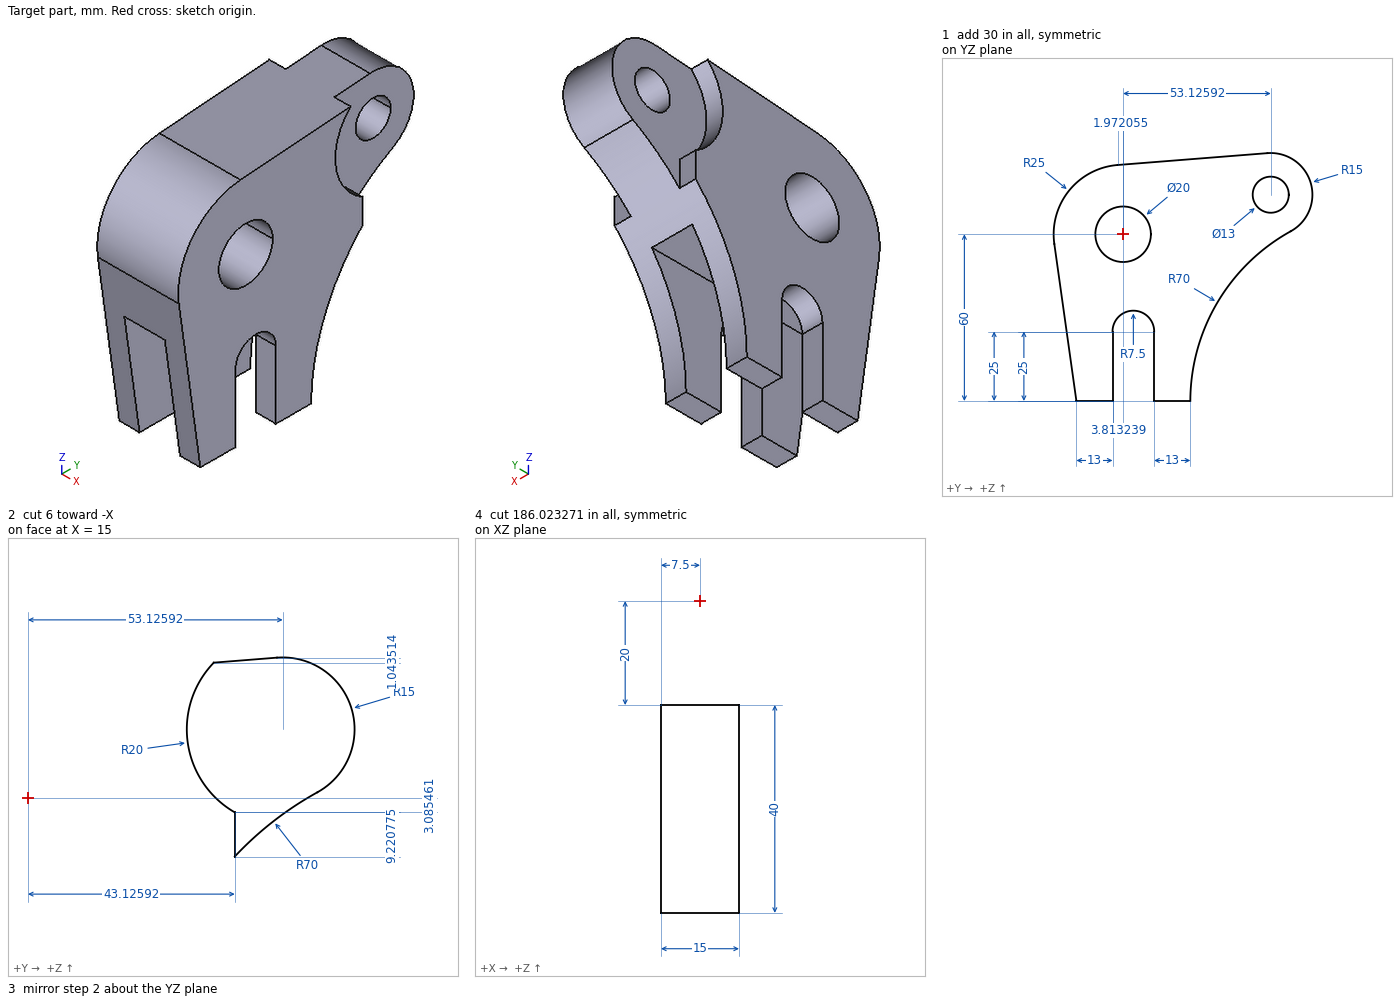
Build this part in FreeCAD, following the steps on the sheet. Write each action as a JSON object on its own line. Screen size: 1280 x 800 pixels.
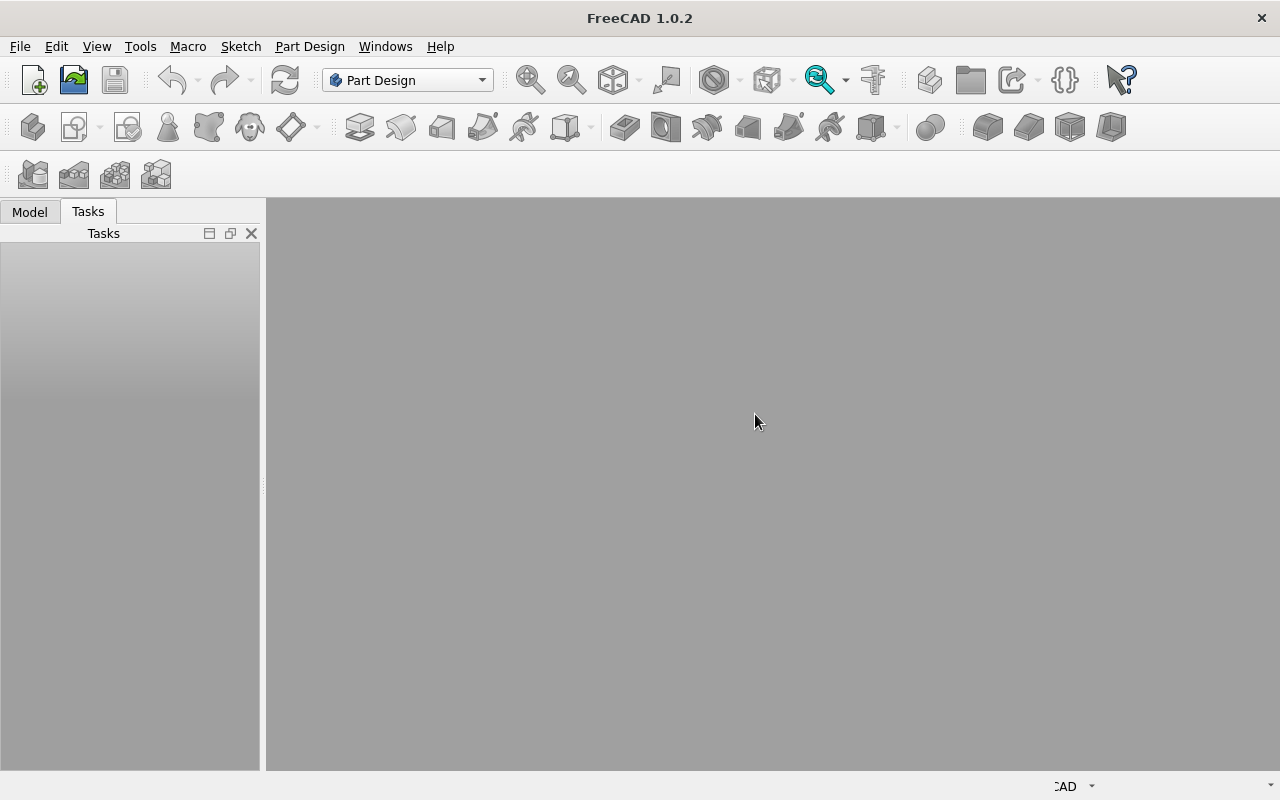
{"action": "left_click", "coordinate": [33, 80]}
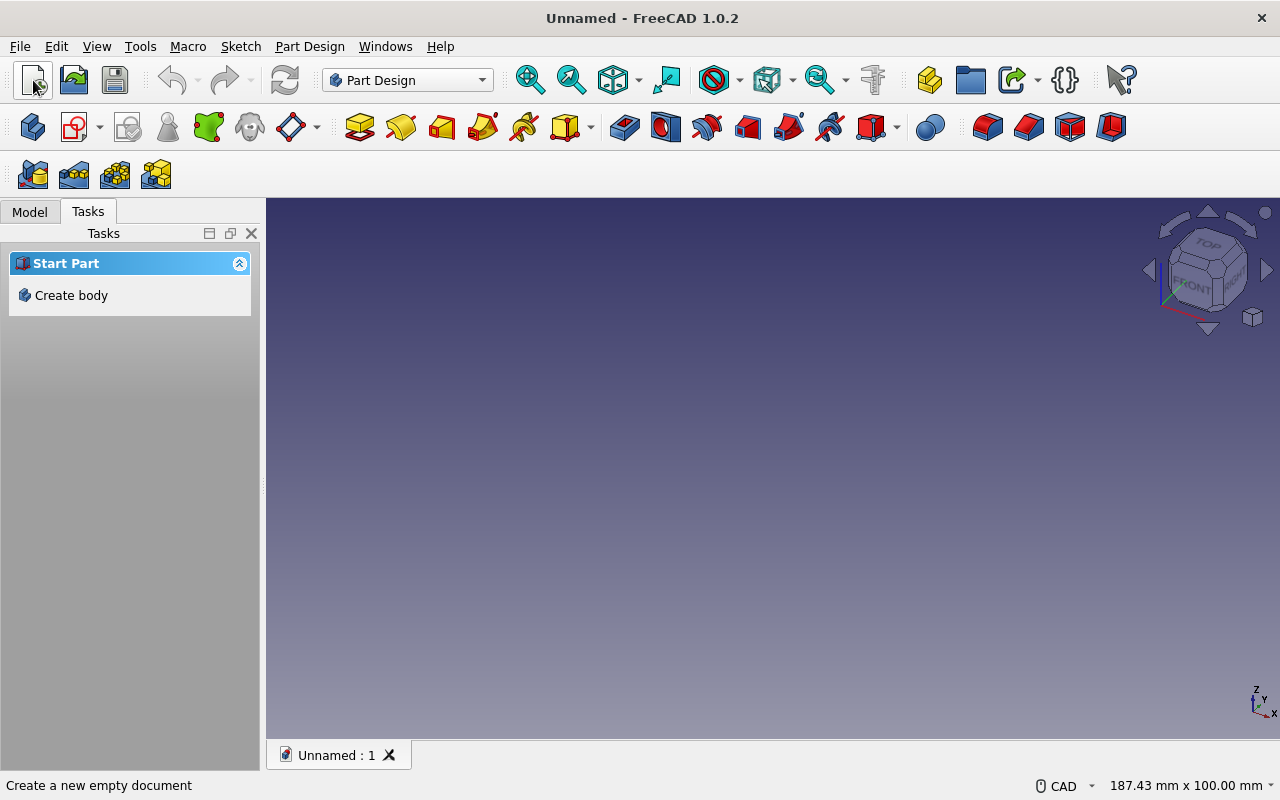
{"action": "left_click", "coordinate": [74, 128]}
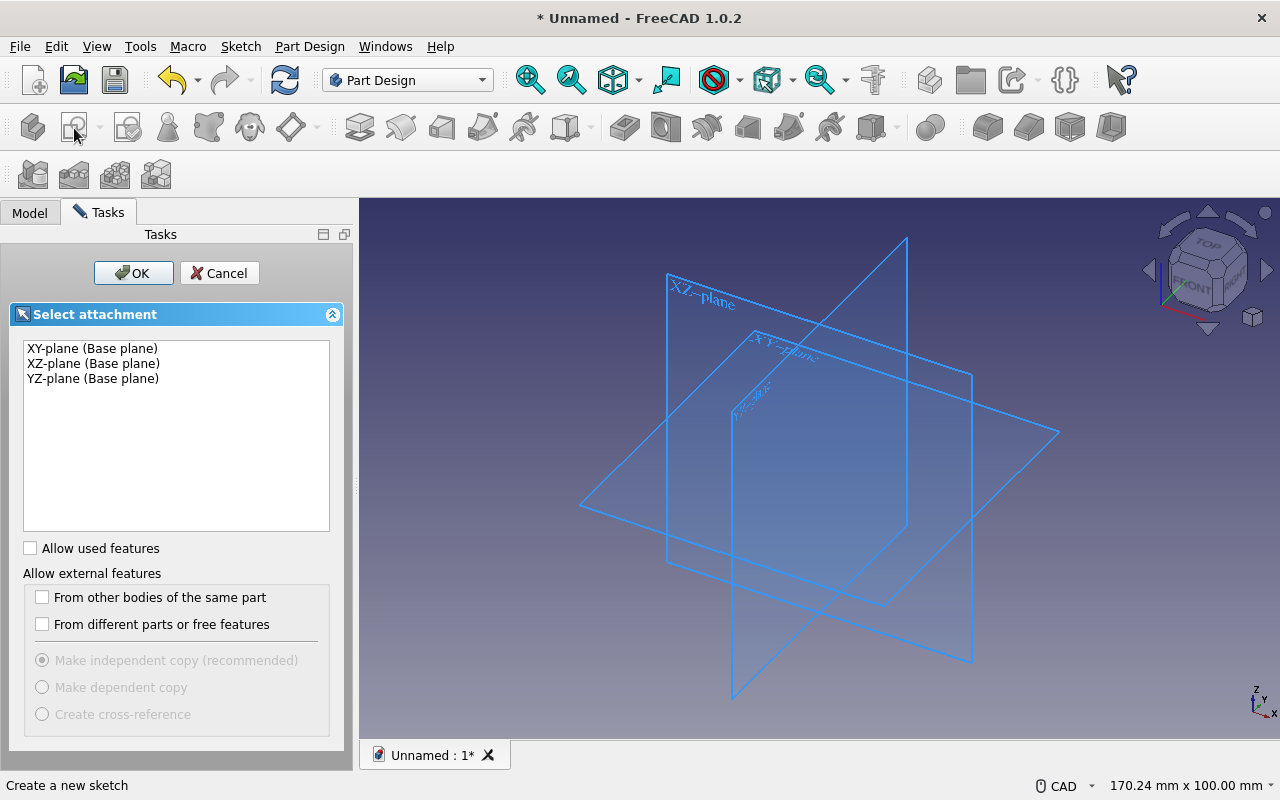
{"action": "left_click", "coordinate": [84, 378]}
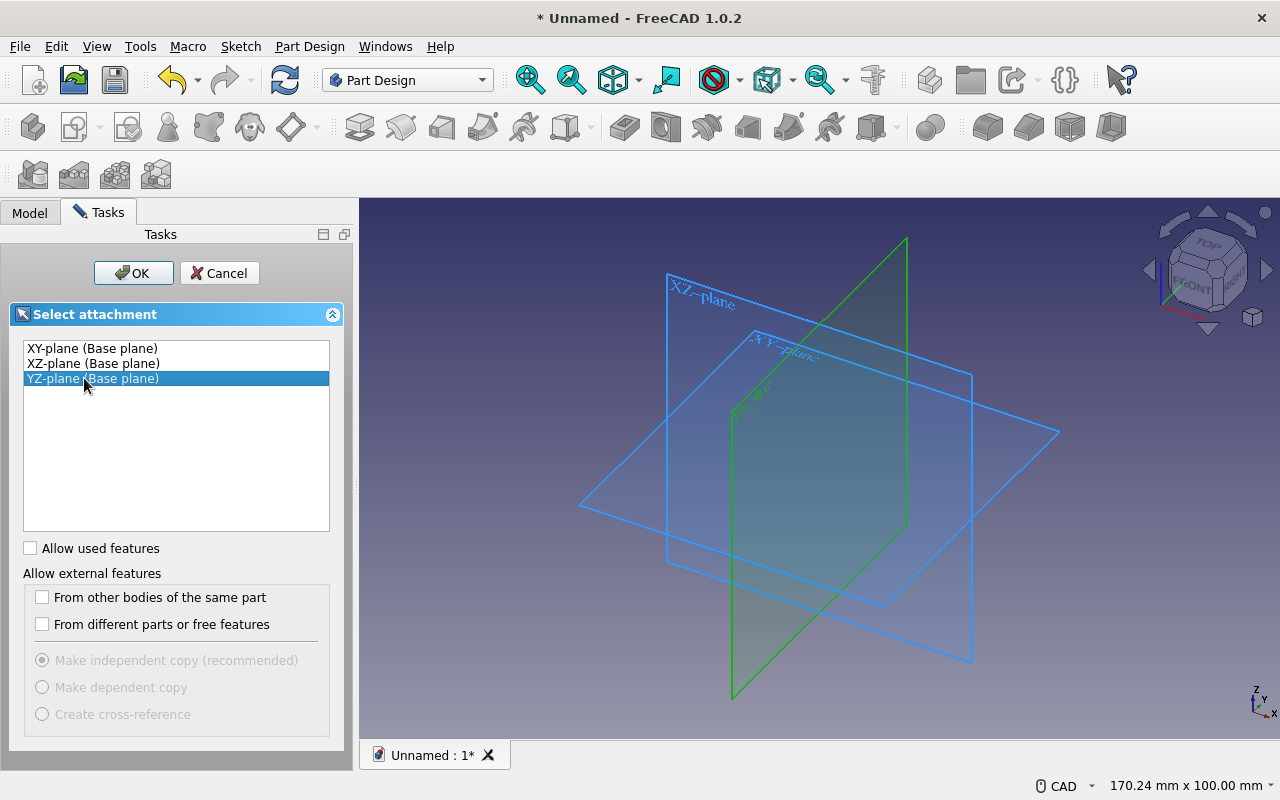
{"action": "left_click", "coordinate": [134, 273]}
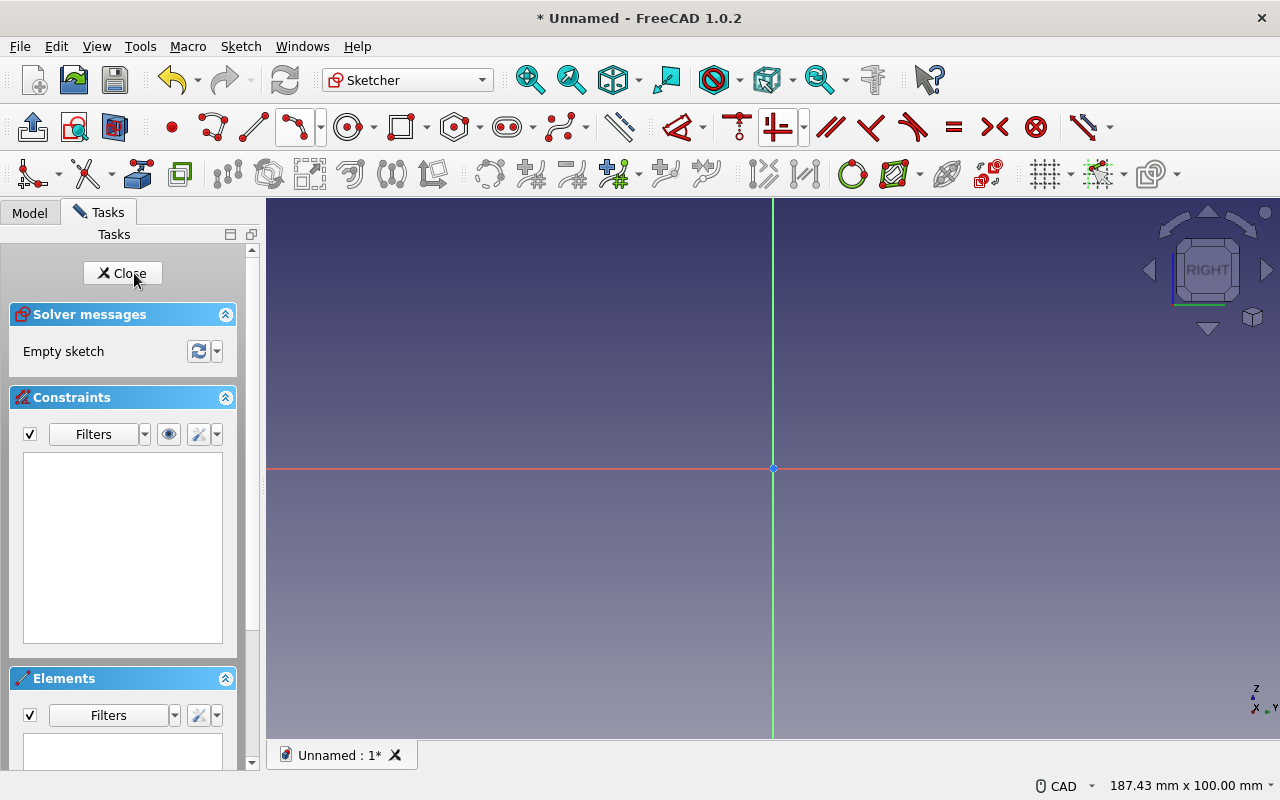
{"action": "scroll", "coordinate": [330, 299], "scroll_direction": "down", "scroll_amount": 2}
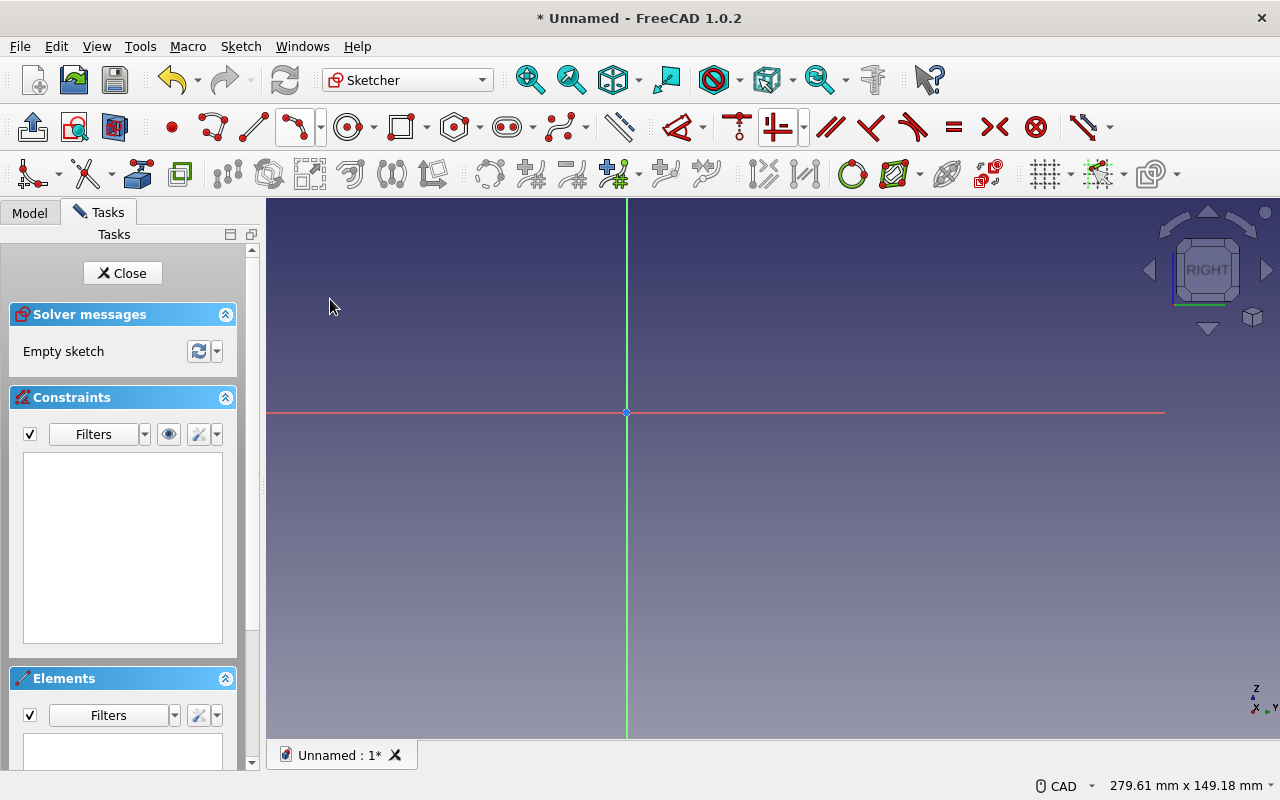
{"action": "left_click", "coordinate": [254, 128]}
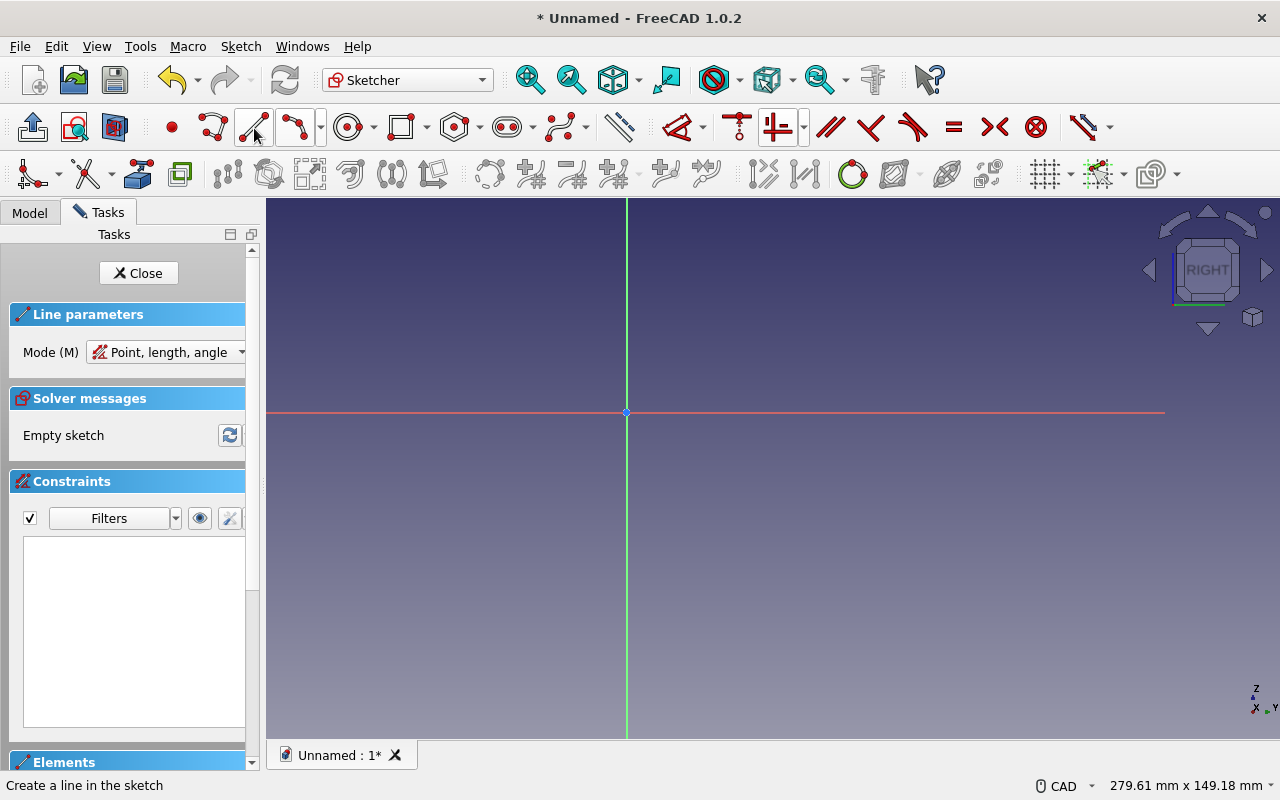
{"action": "left_click", "coordinate": [815, 307]}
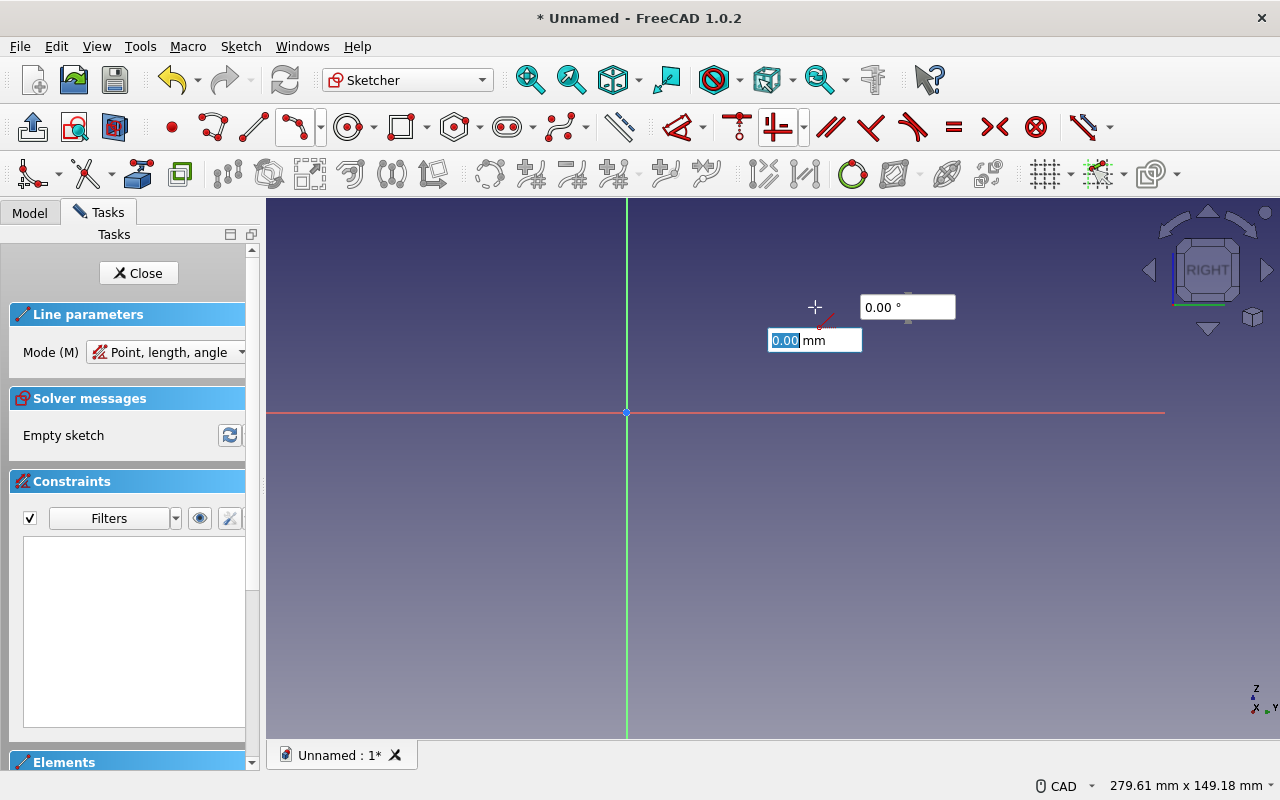
{"action": "scroll", "coordinate": [620, 322], "scroll_direction": "up", "scroll_amount": 4}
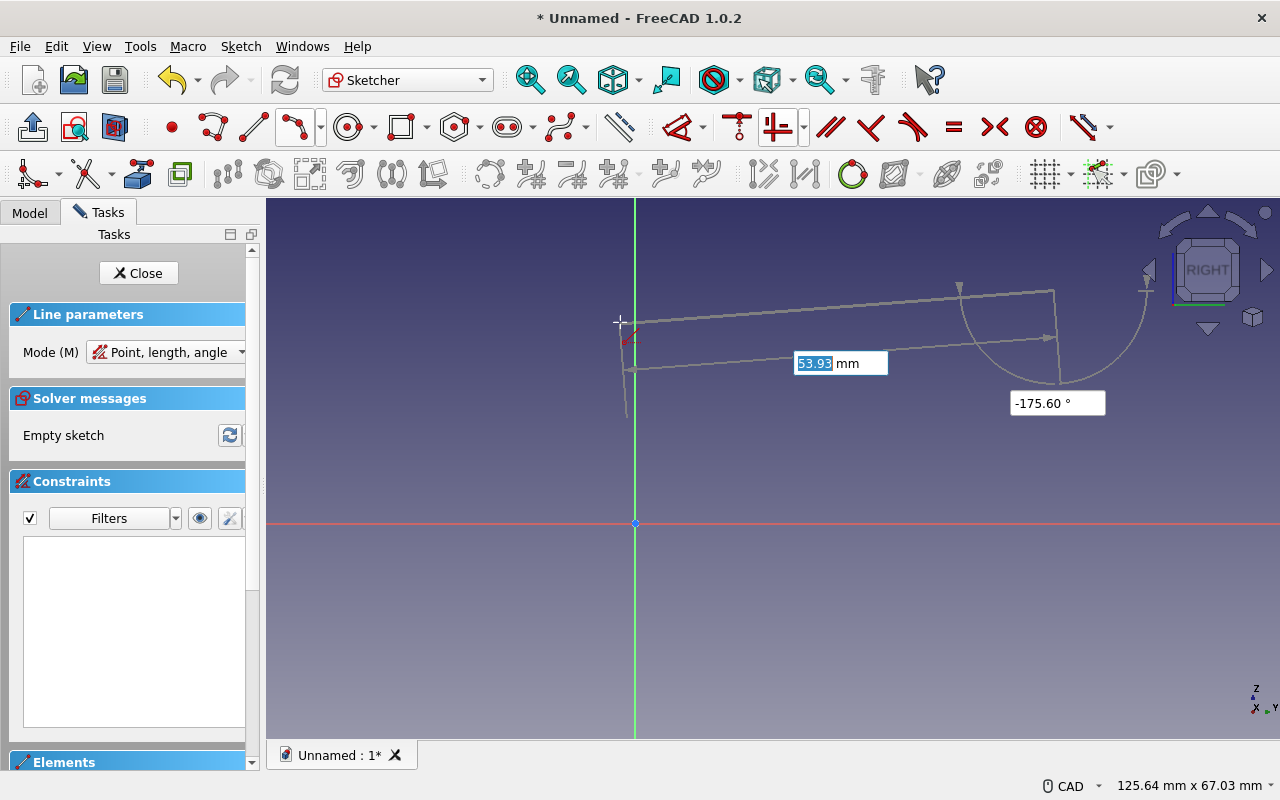
{"action": "left_click", "coordinate": [619, 322]}